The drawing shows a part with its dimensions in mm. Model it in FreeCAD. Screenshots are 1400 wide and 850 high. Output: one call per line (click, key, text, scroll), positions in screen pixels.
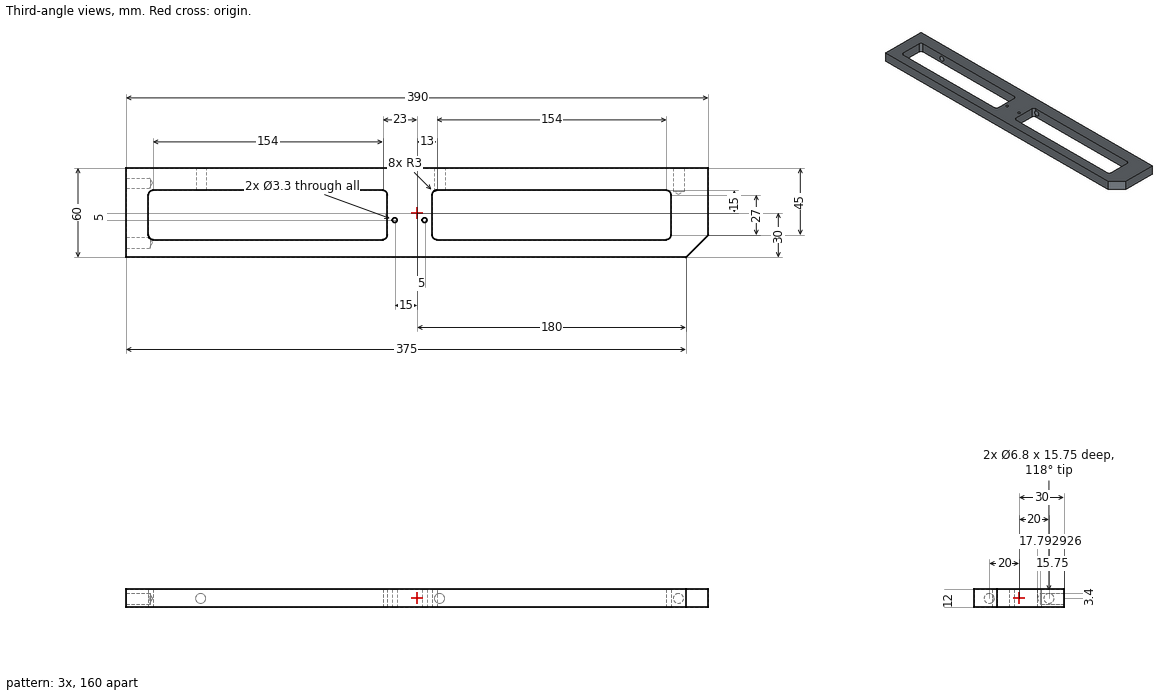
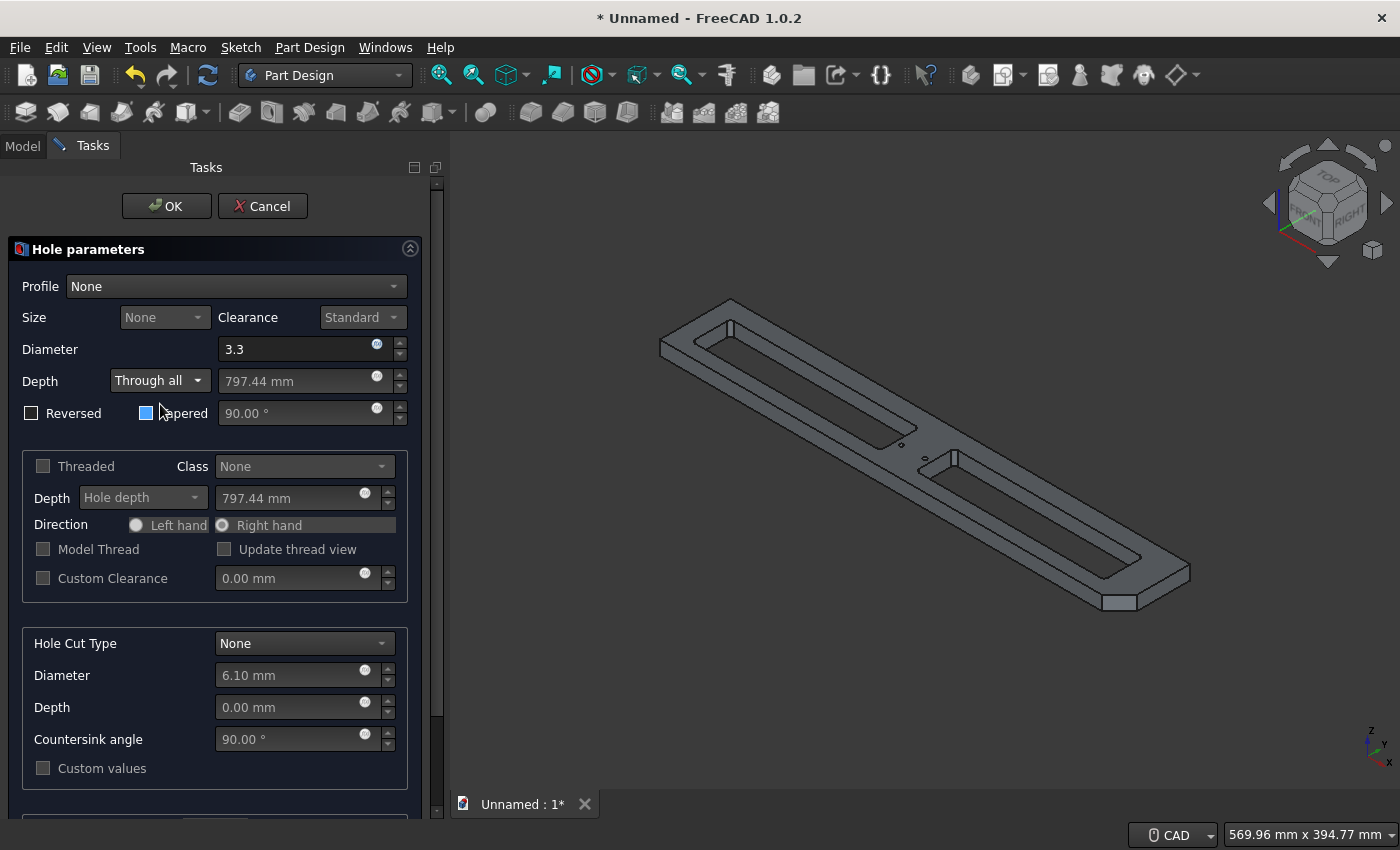
click(167, 206)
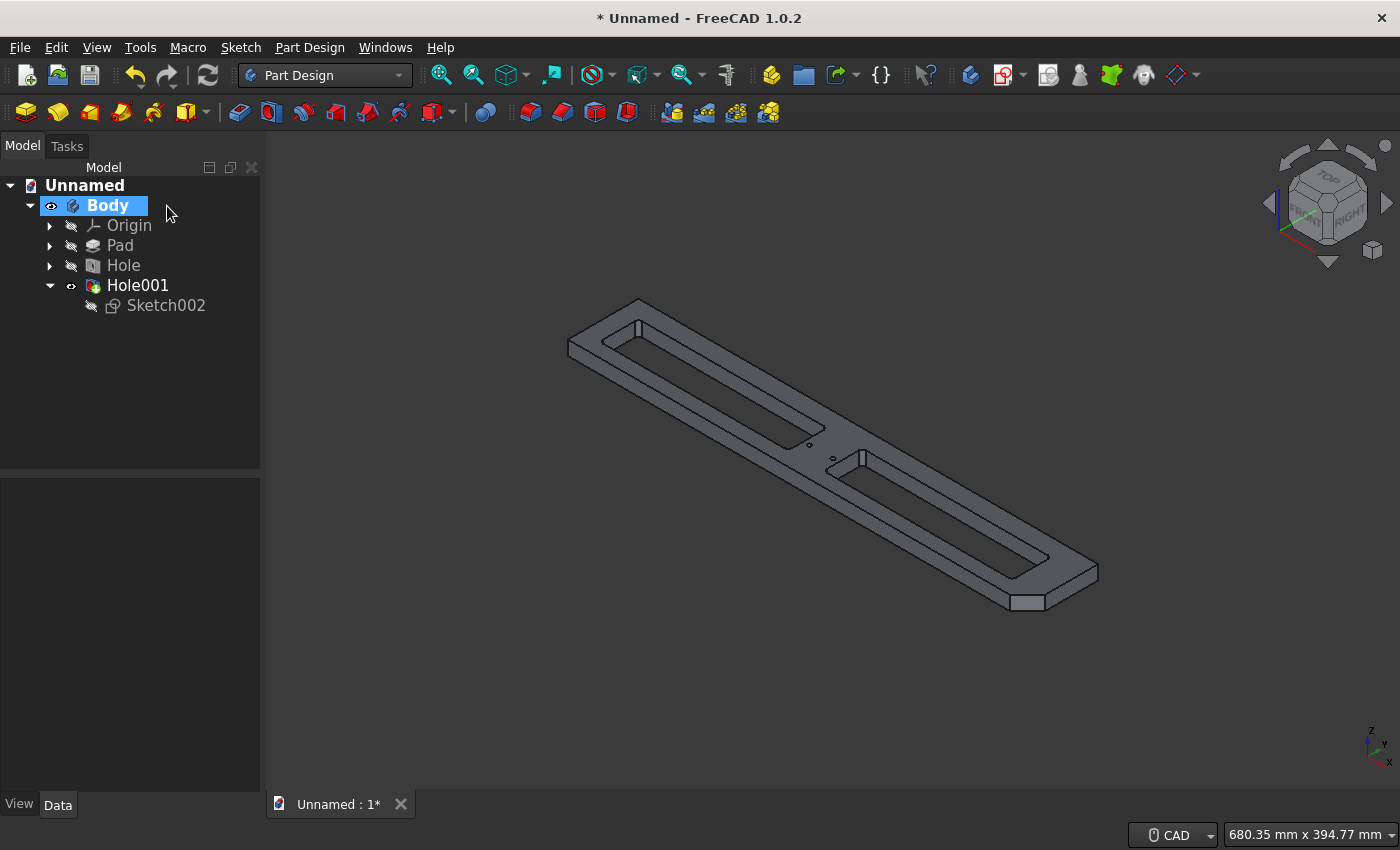
click(50, 226)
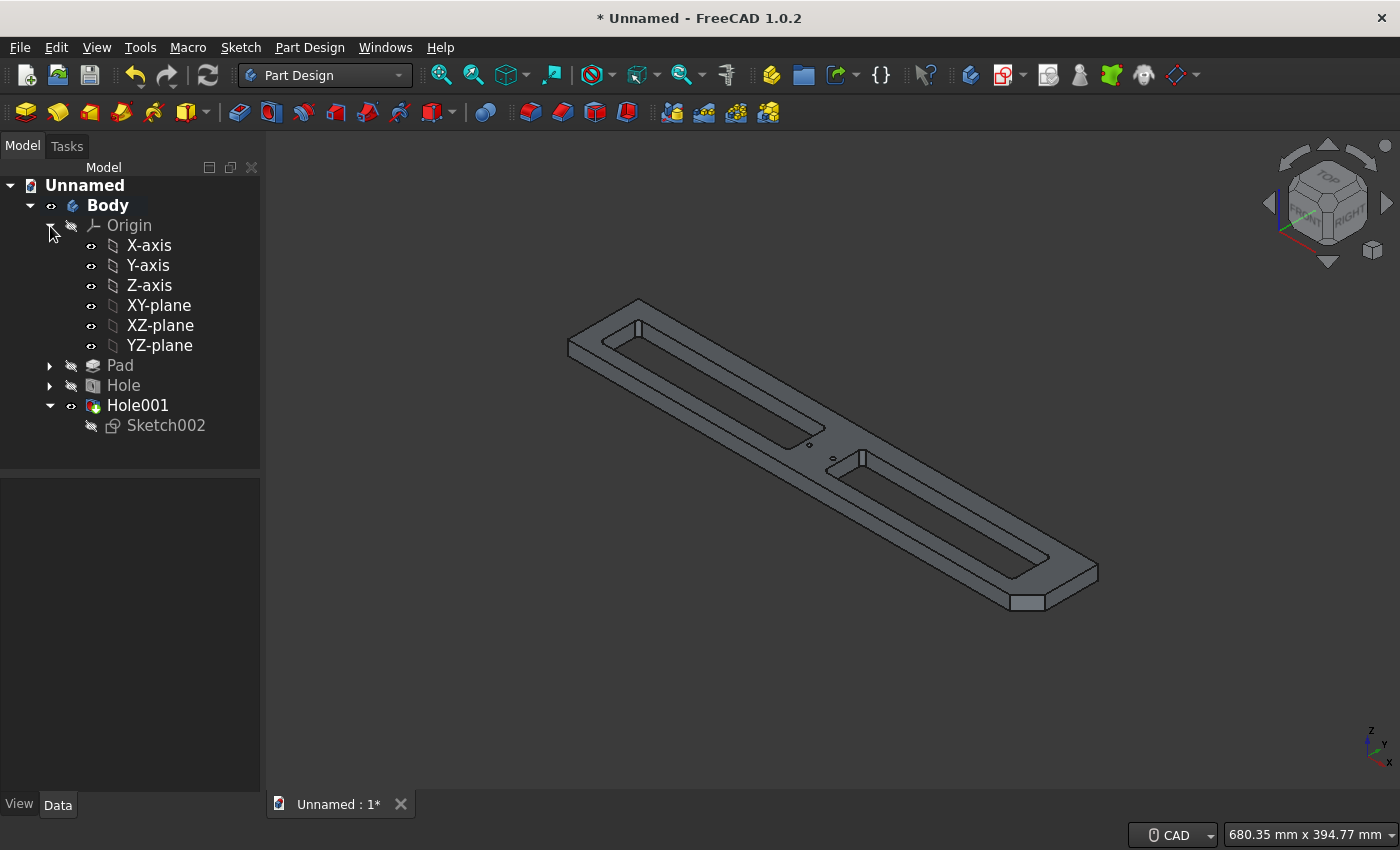
click(136, 346)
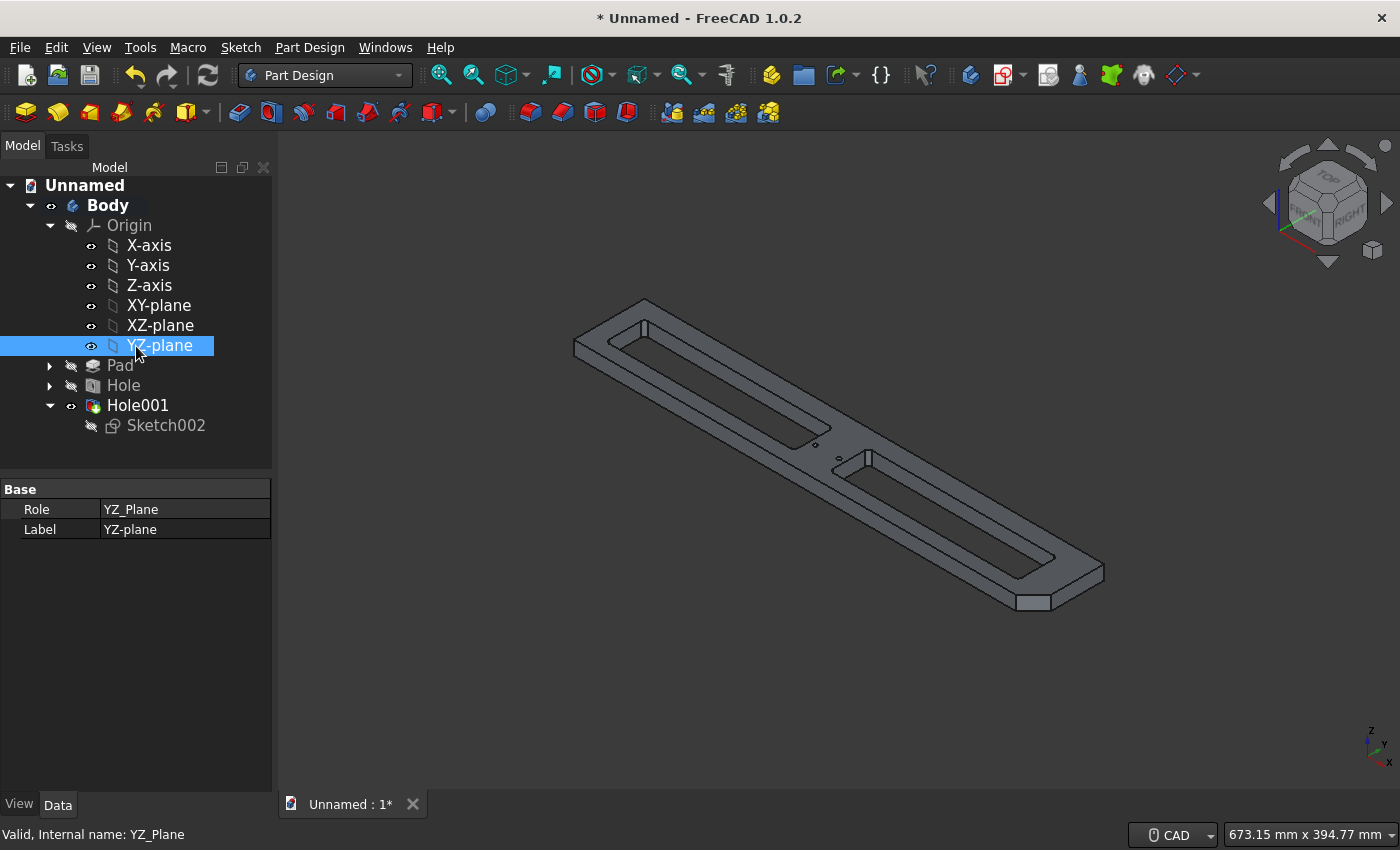
click(1176, 76)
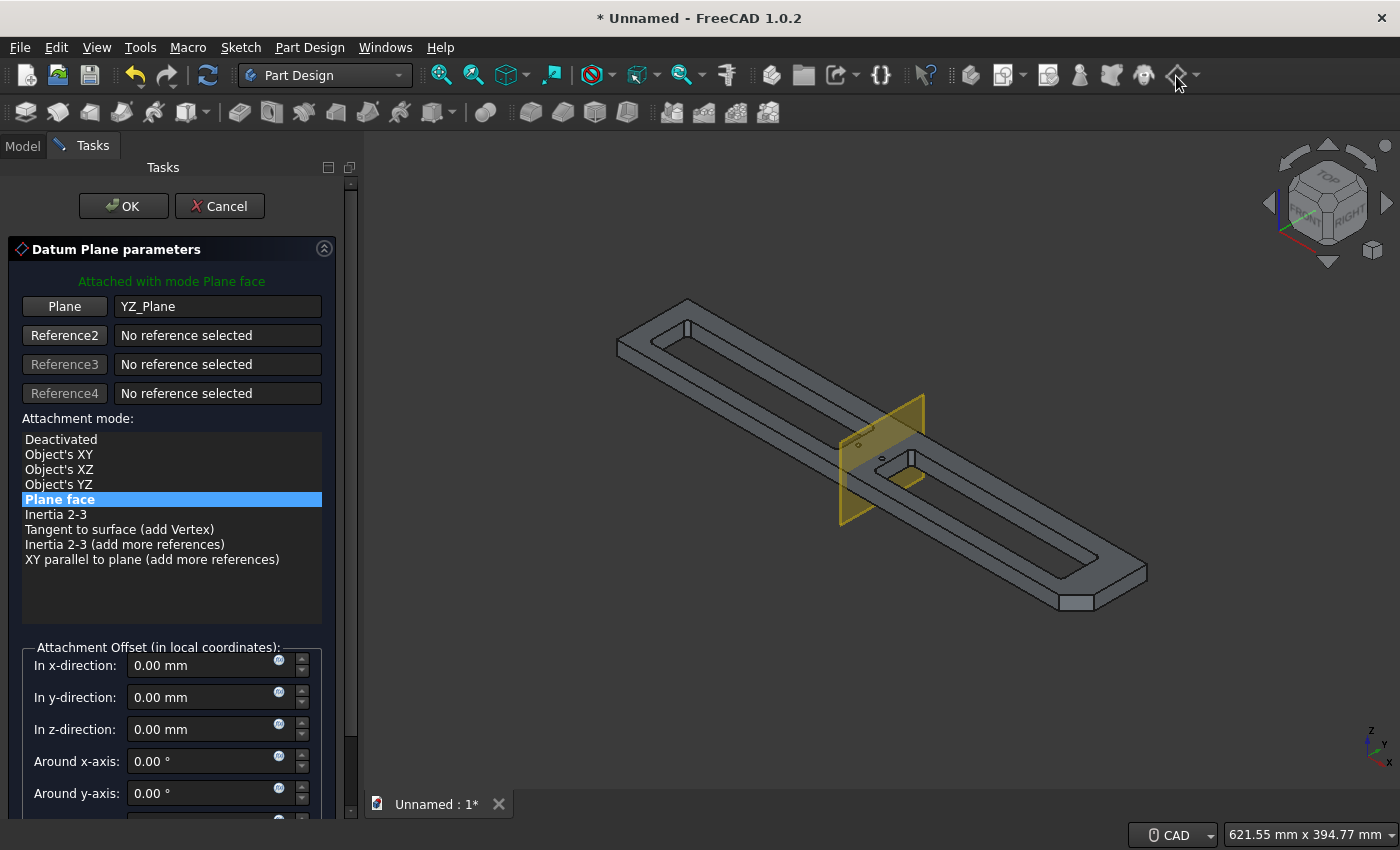
triple_click(210, 729)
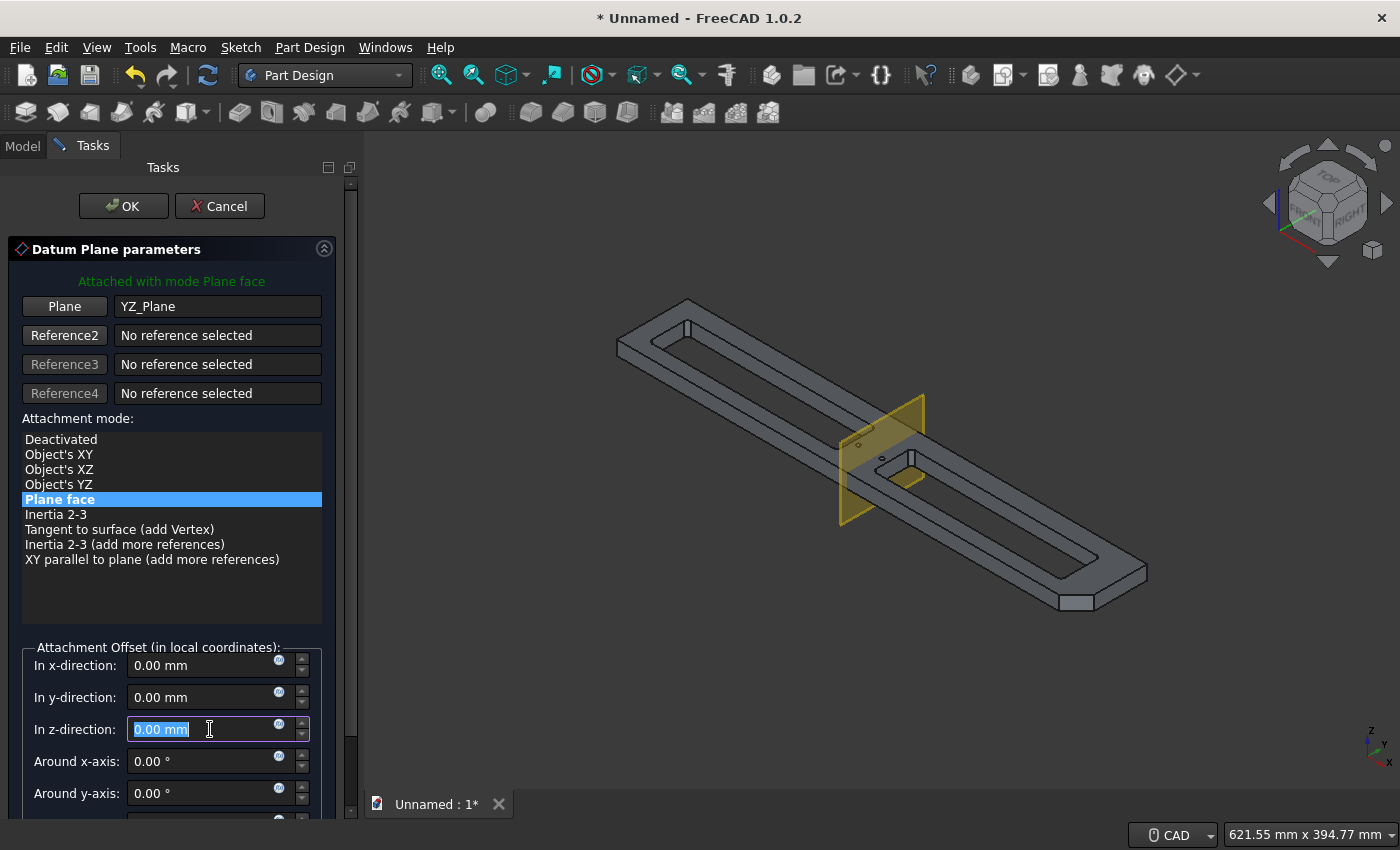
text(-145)
key(Tab)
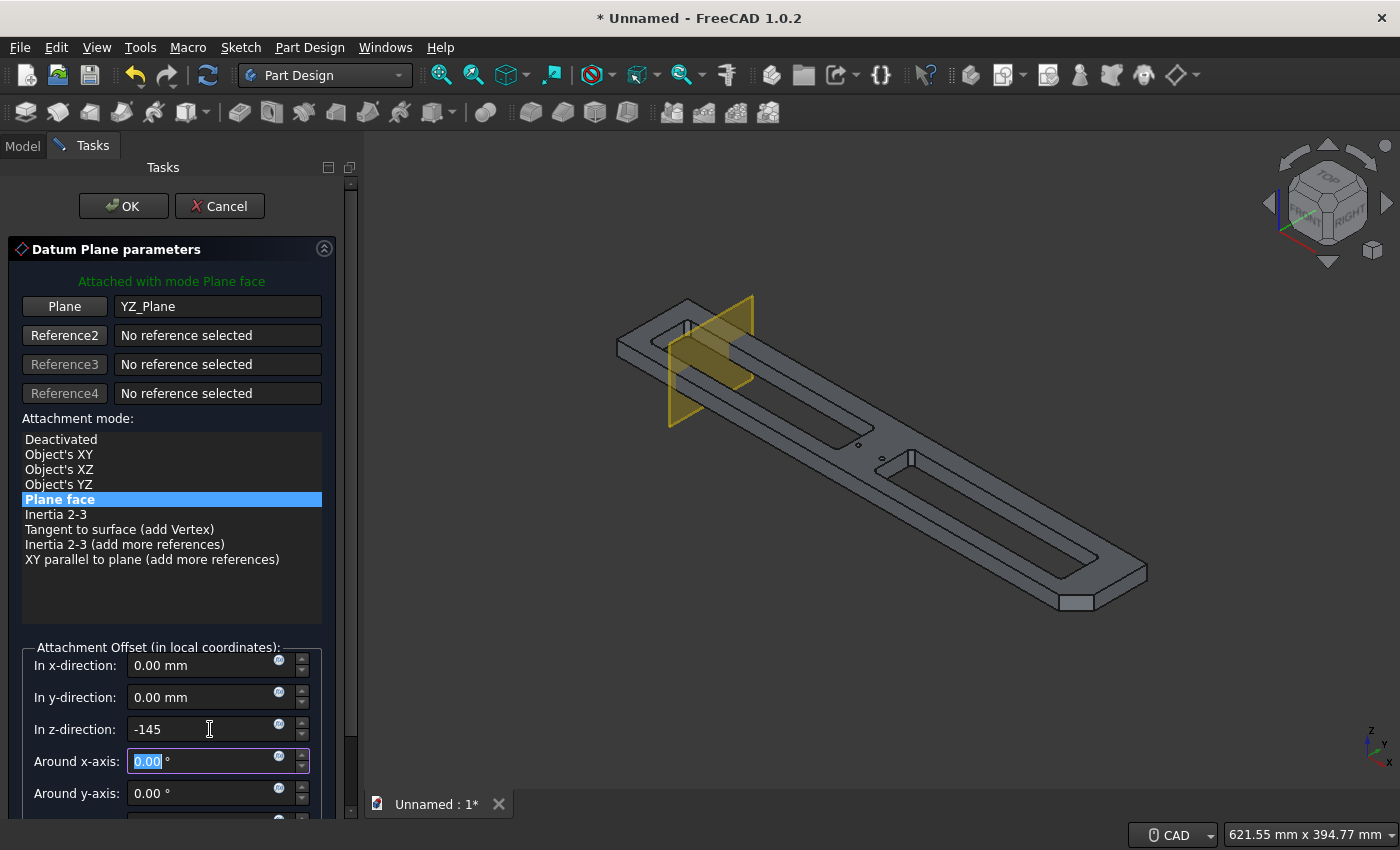
click(124, 206)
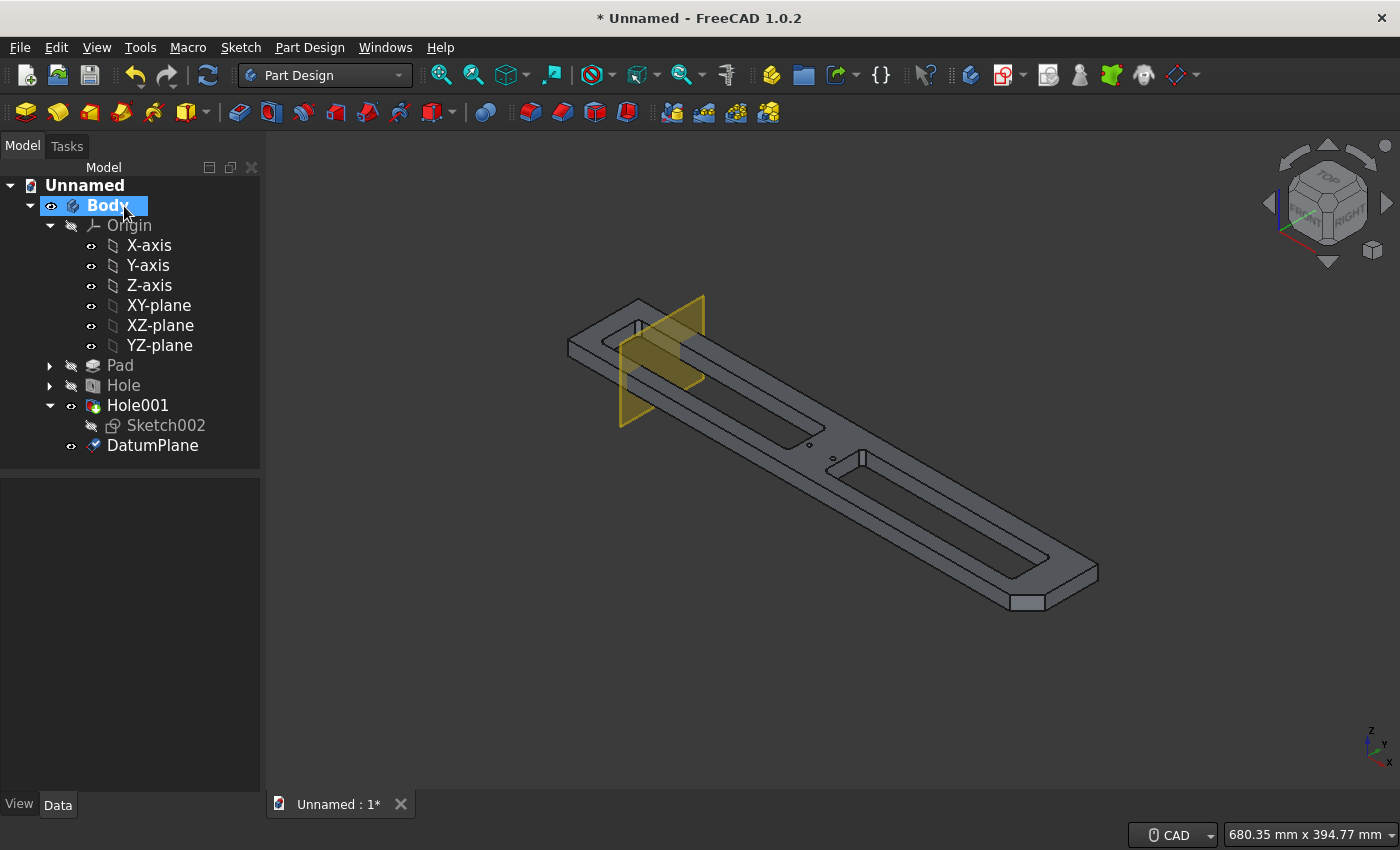
click(116, 446)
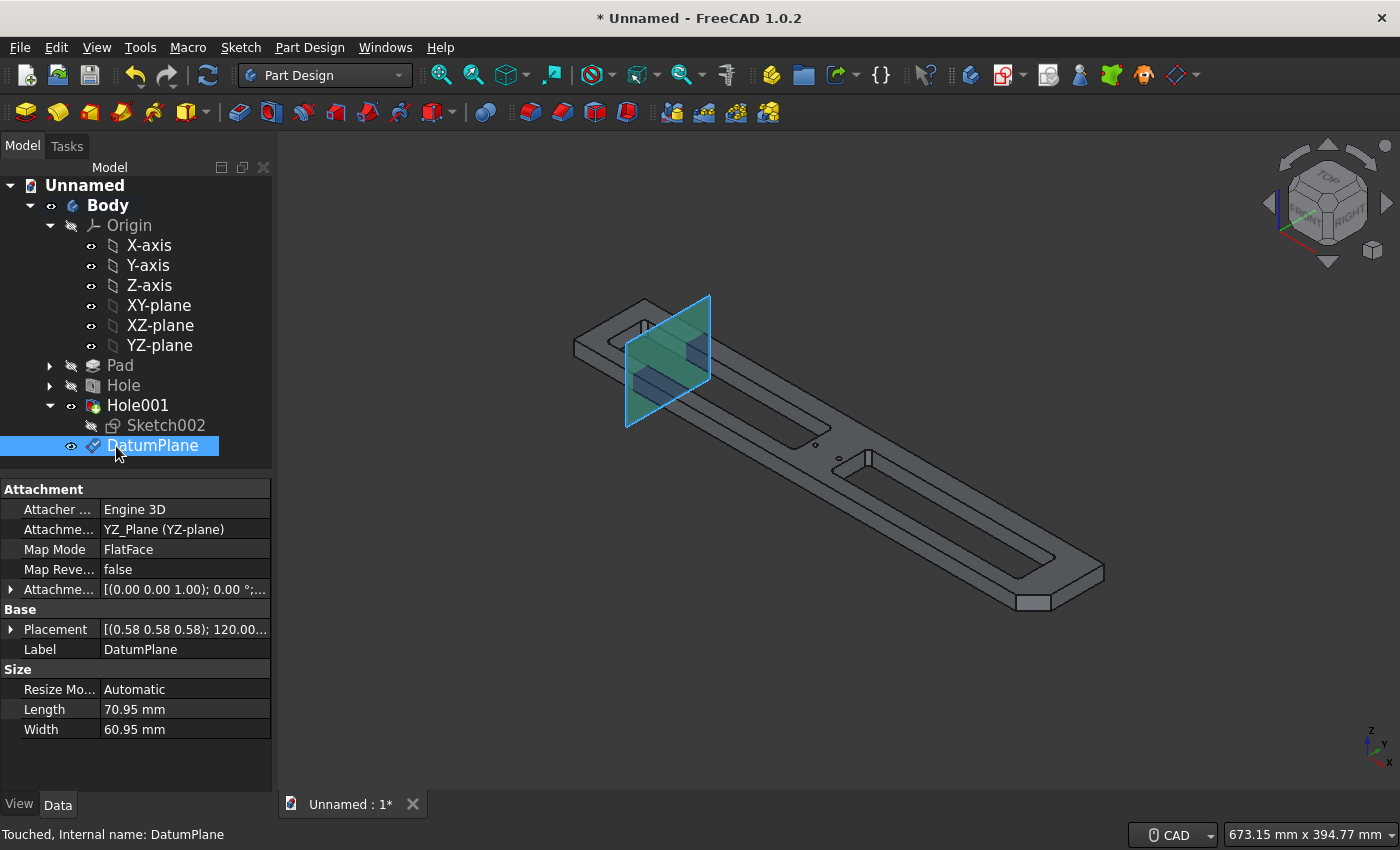
click(1004, 76)